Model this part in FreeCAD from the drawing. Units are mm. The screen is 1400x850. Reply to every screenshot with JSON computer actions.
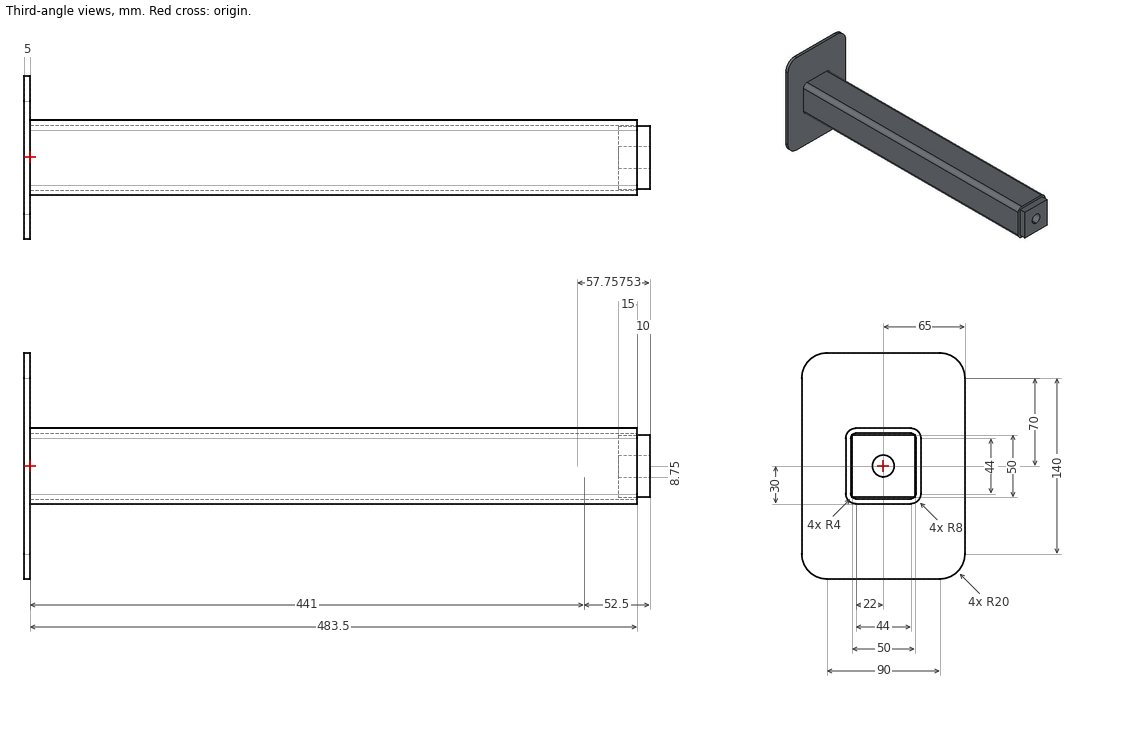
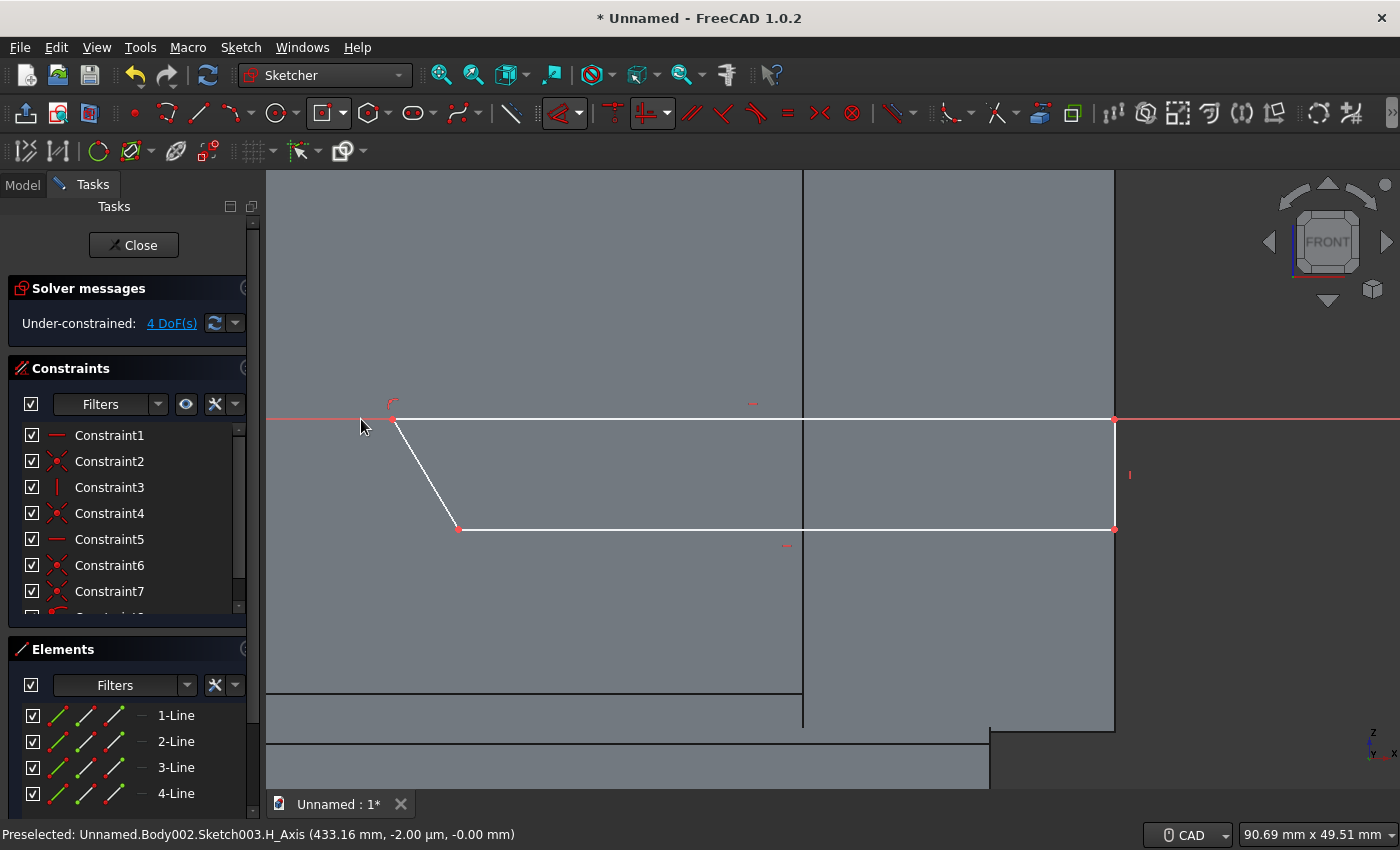
{"action": "left_click", "coordinate": [1115, 452]}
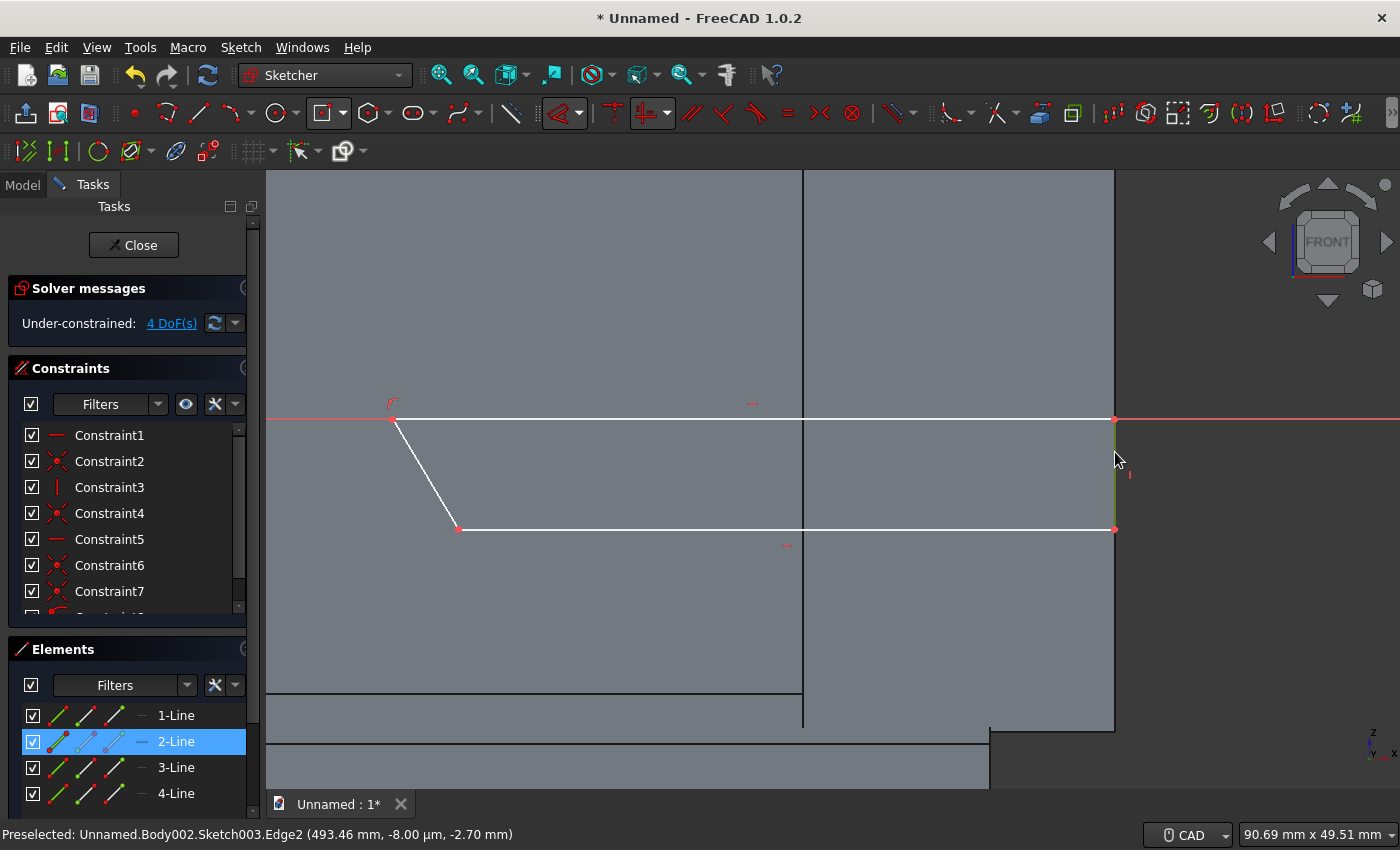
{"action": "left_click", "coordinate": [582, 114]}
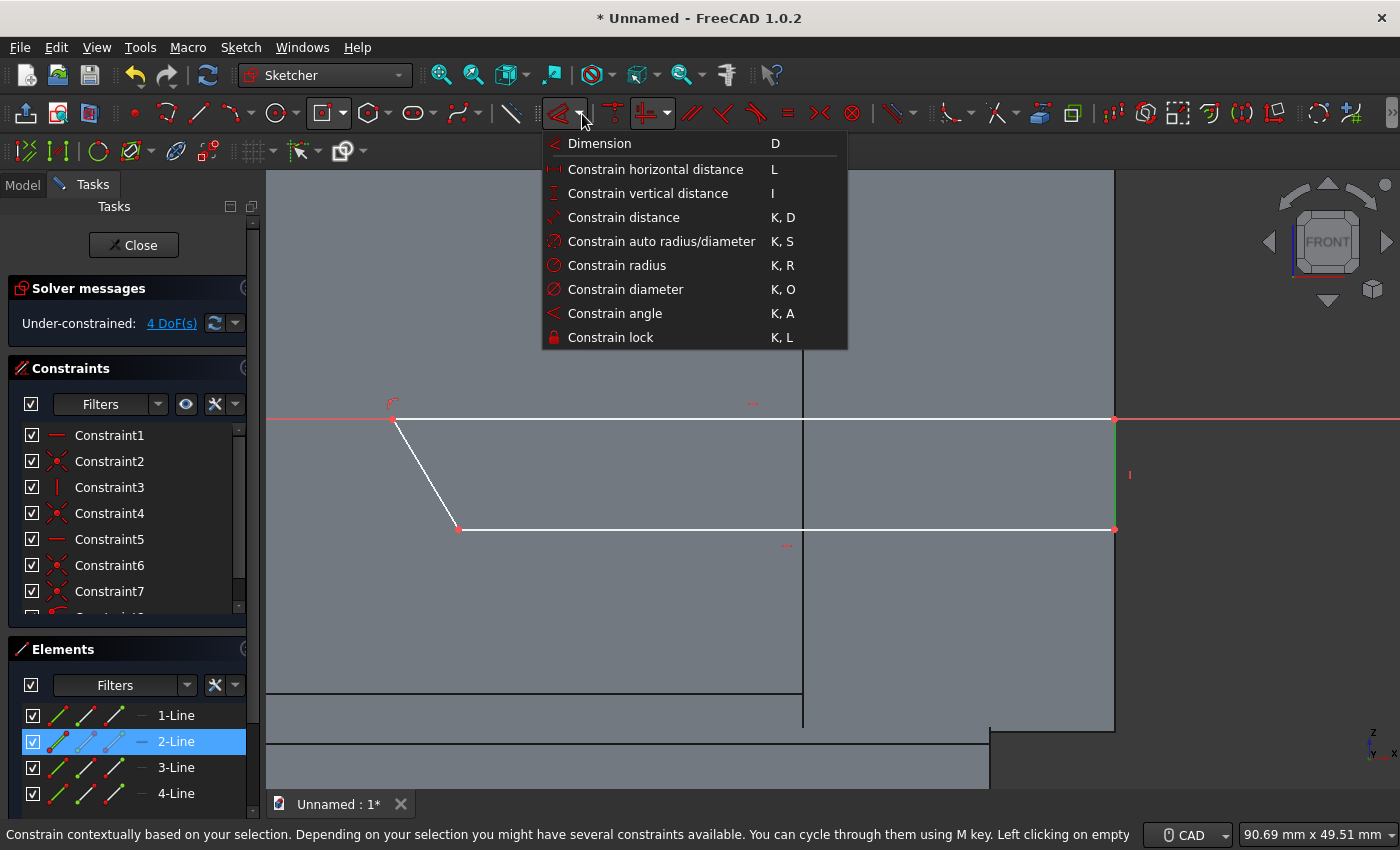
{"action": "left_click", "coordinate": [695, 193]}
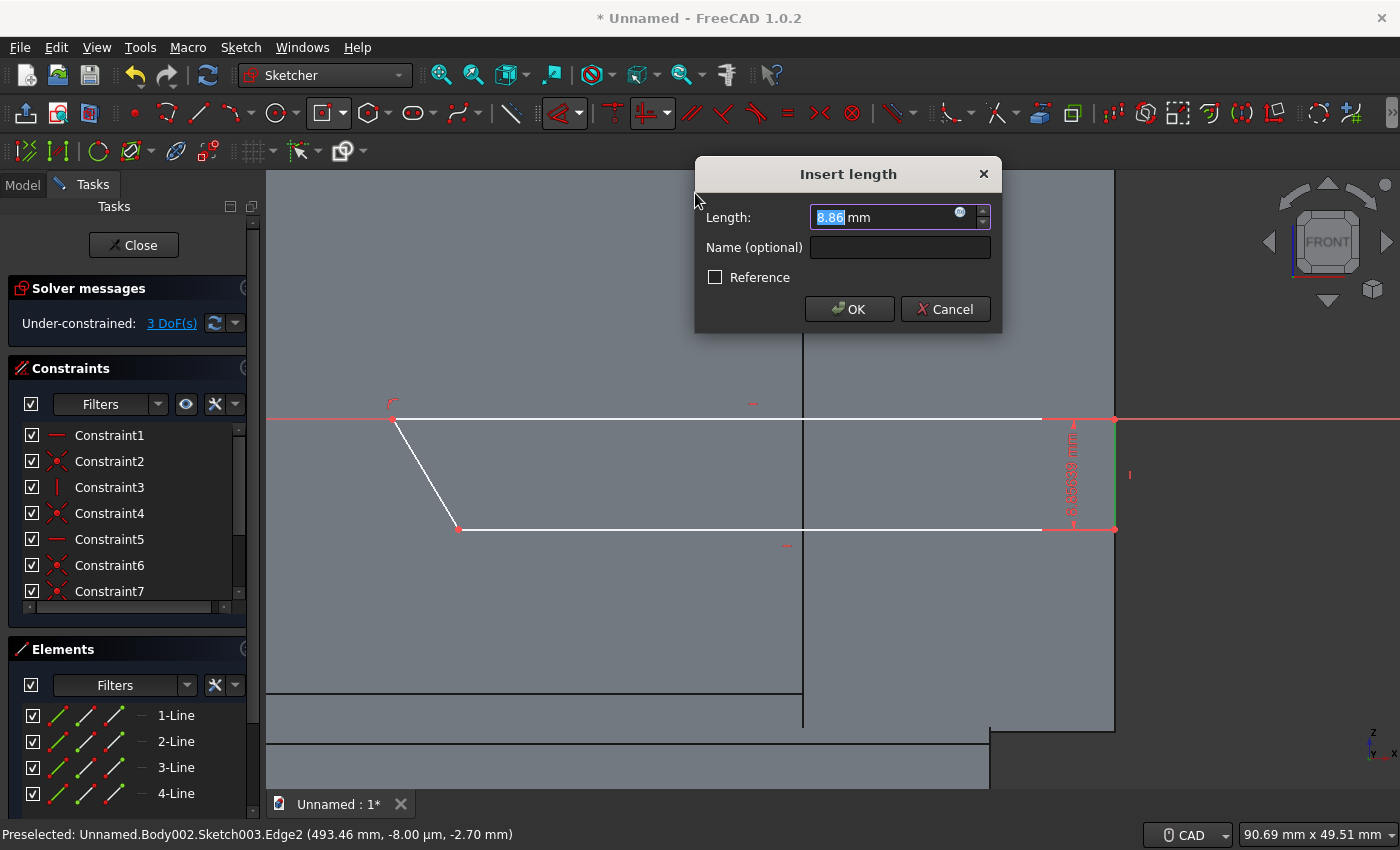
{"action": "type", "text": "8.75"}
{"action": "key", "text": "Return"}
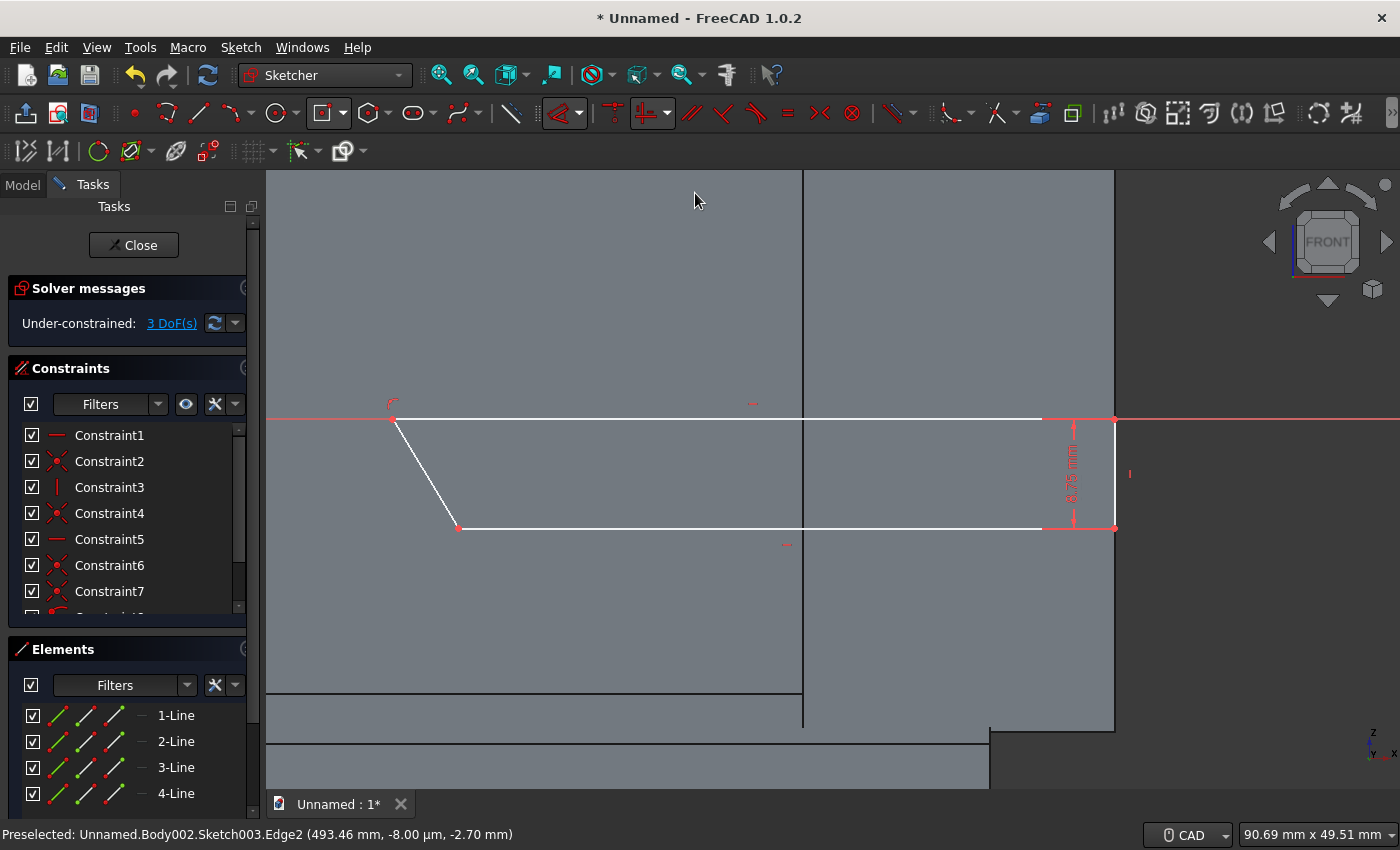
{"action": "left_click", "coordinate": [918, 529]}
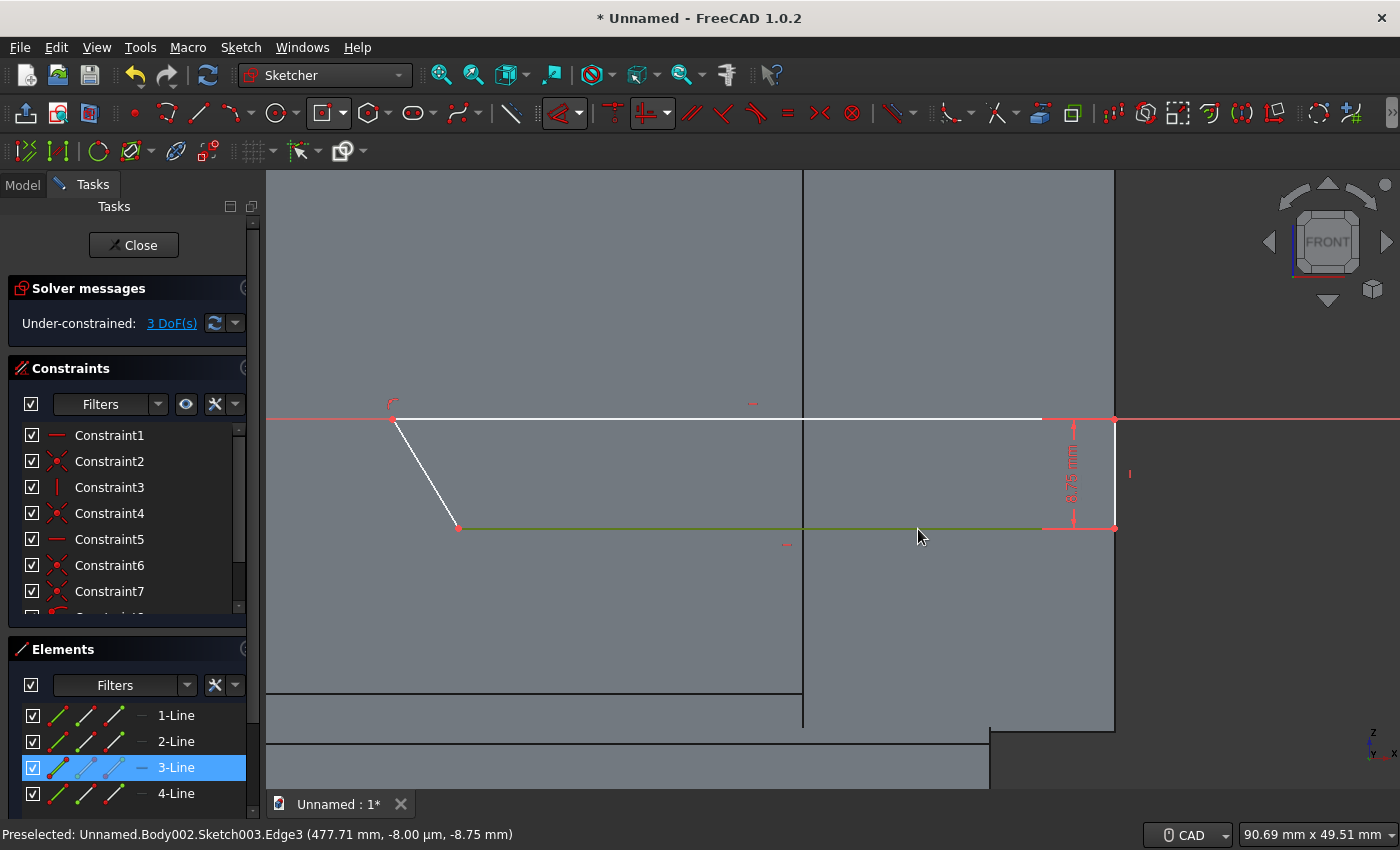
{"action": "key", "text": "l"}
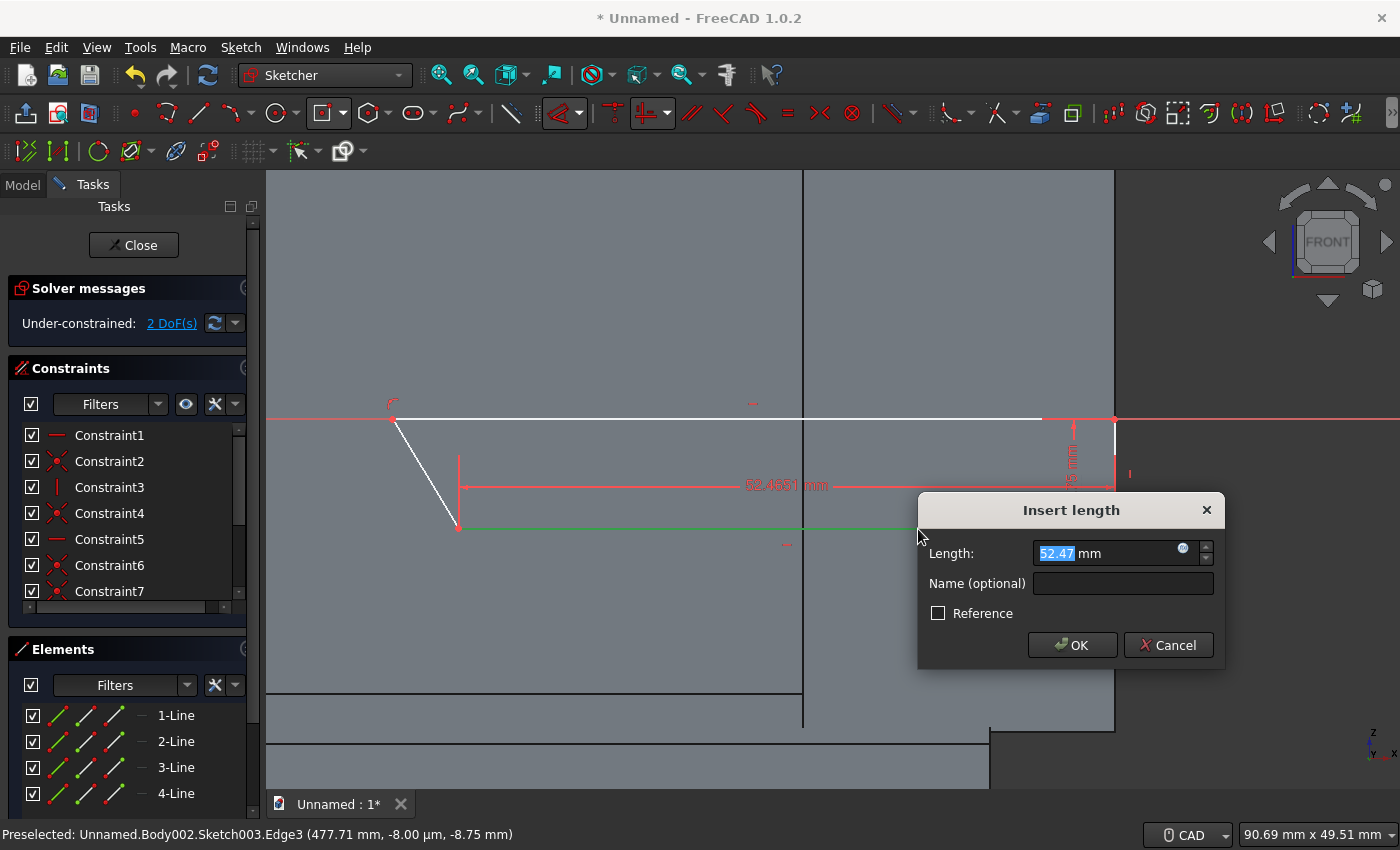
{"action": "type", "text": "52.5"}
{"action": "key", "text": "Return"}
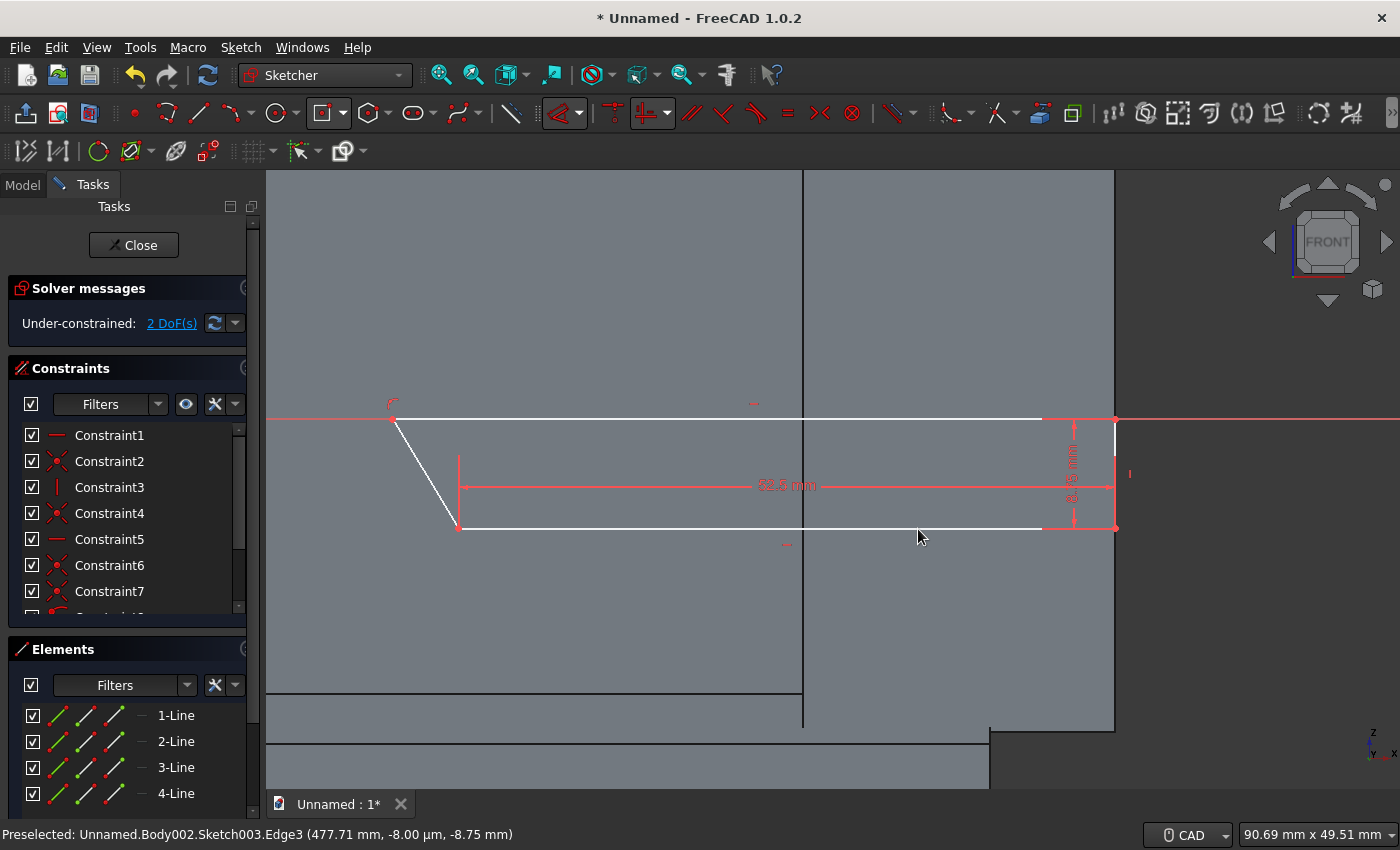
{"action": "left_click", "coordinate": [459, 529]}